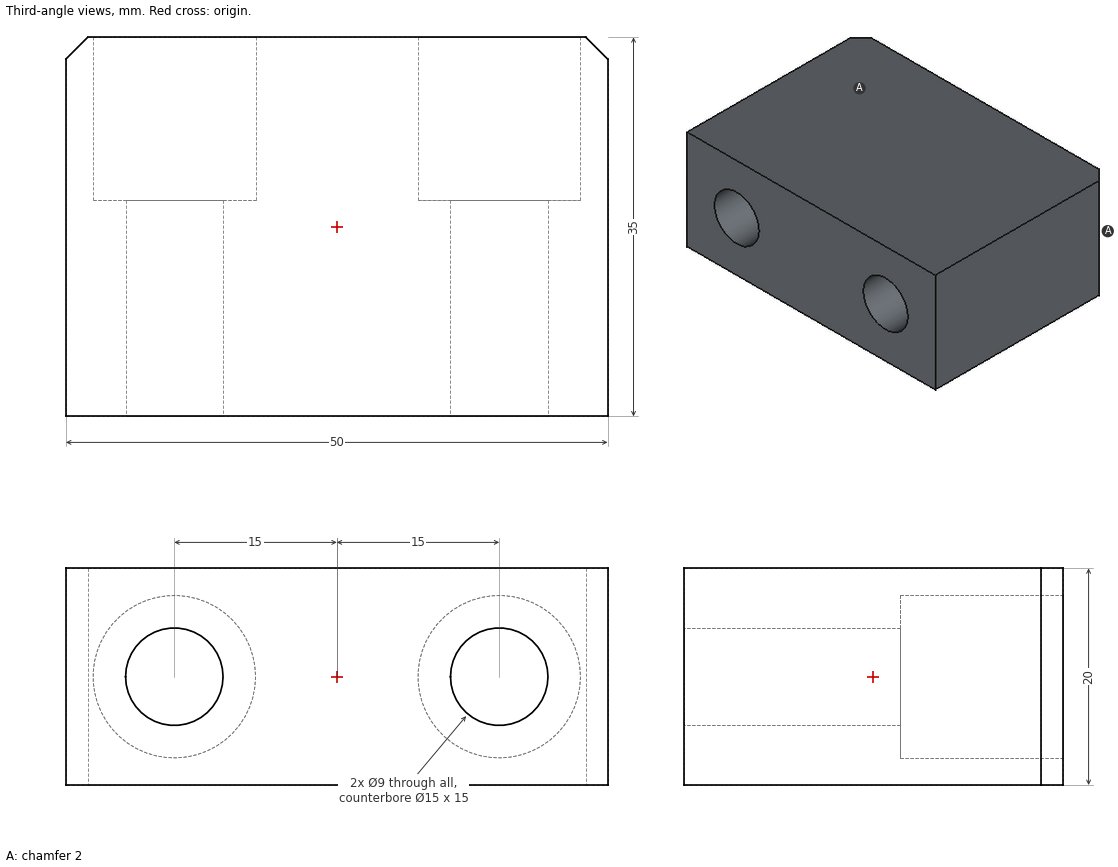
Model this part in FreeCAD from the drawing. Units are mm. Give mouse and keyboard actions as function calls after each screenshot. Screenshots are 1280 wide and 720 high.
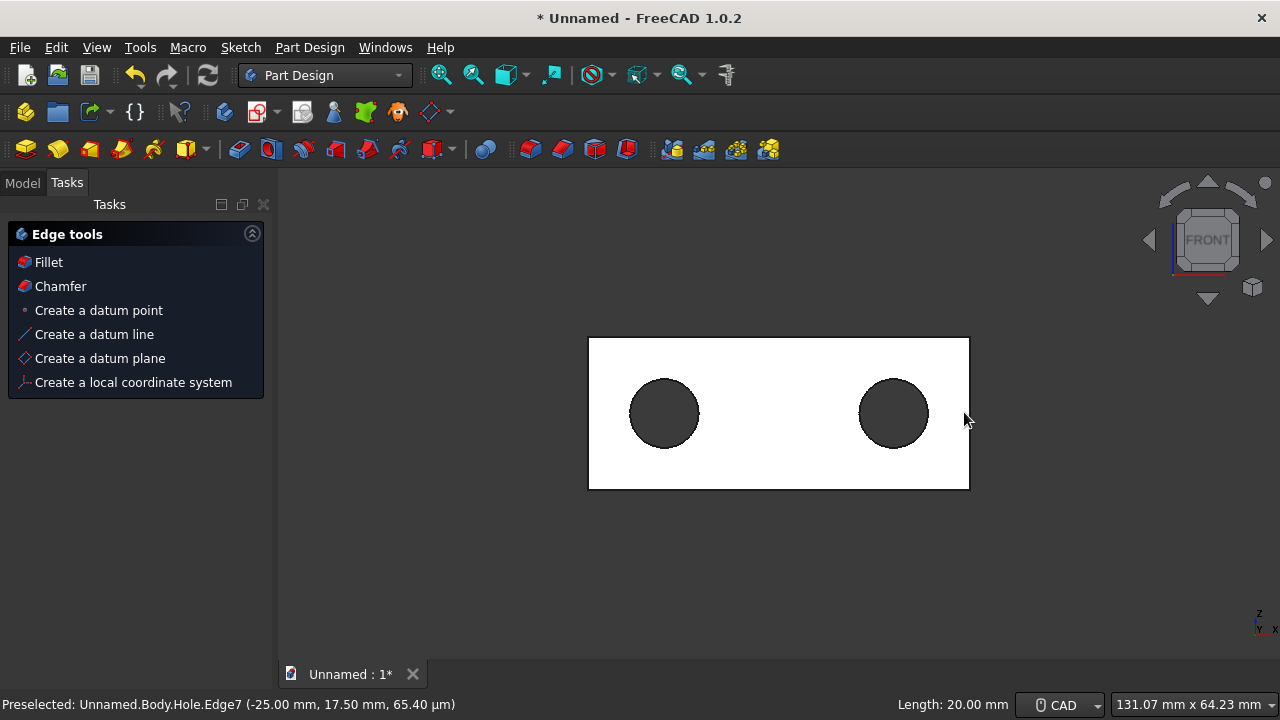
click(442, 76)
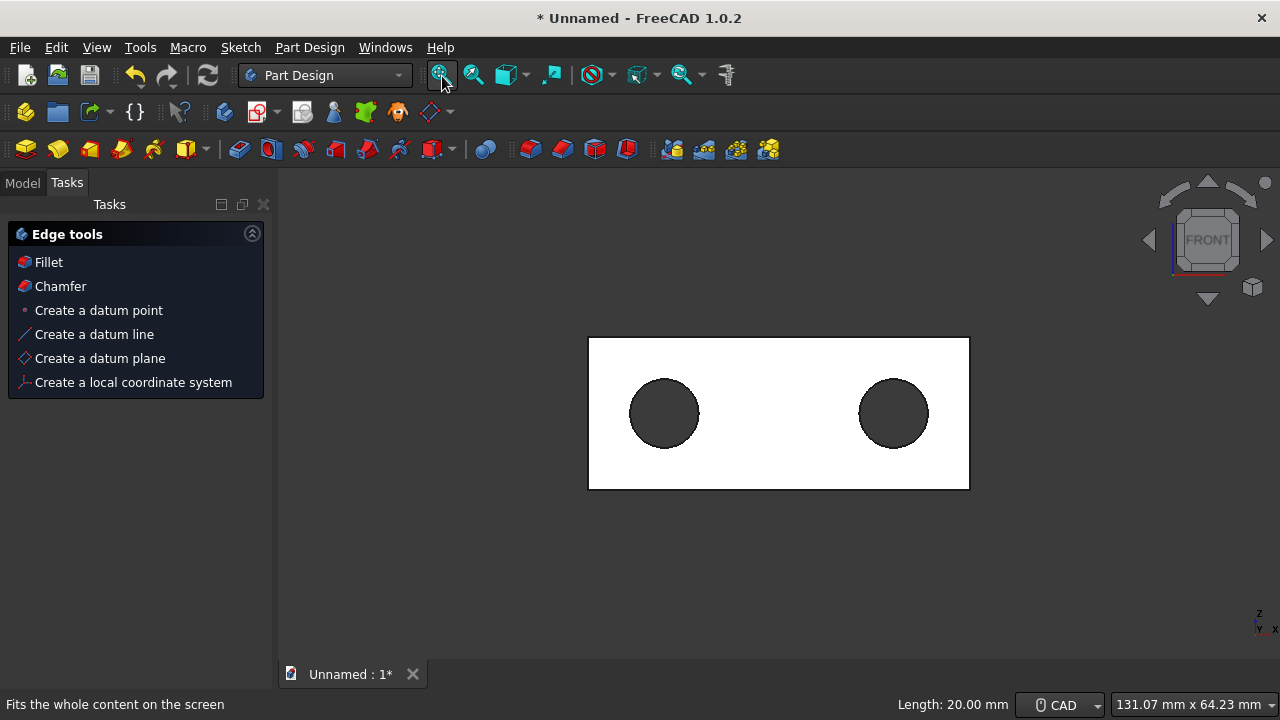
key(3)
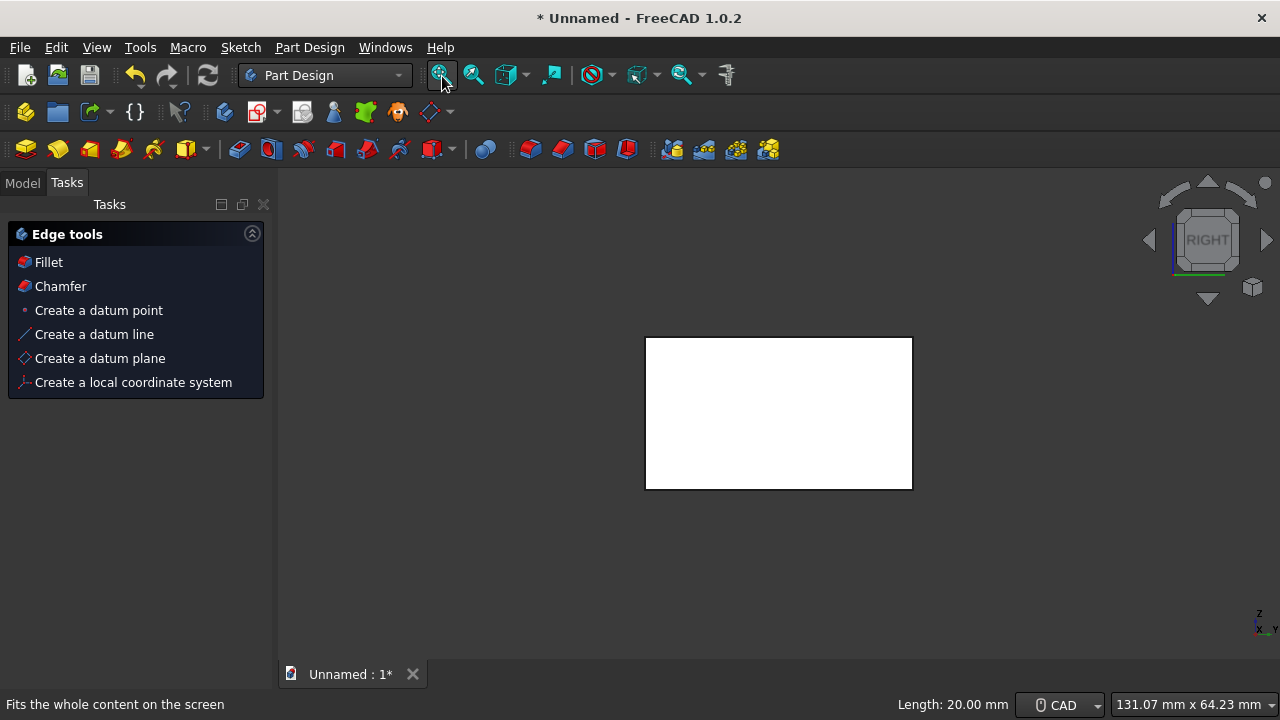
click(442, 76)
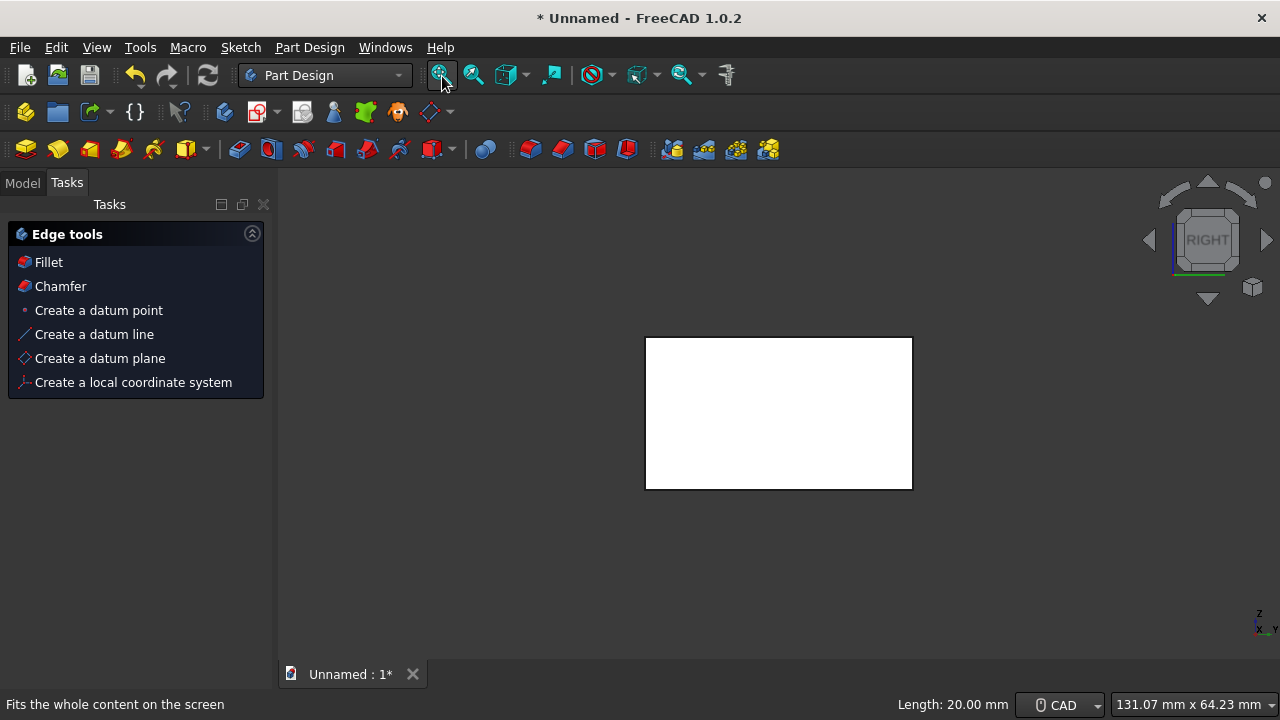
click(913, 412, ctrl)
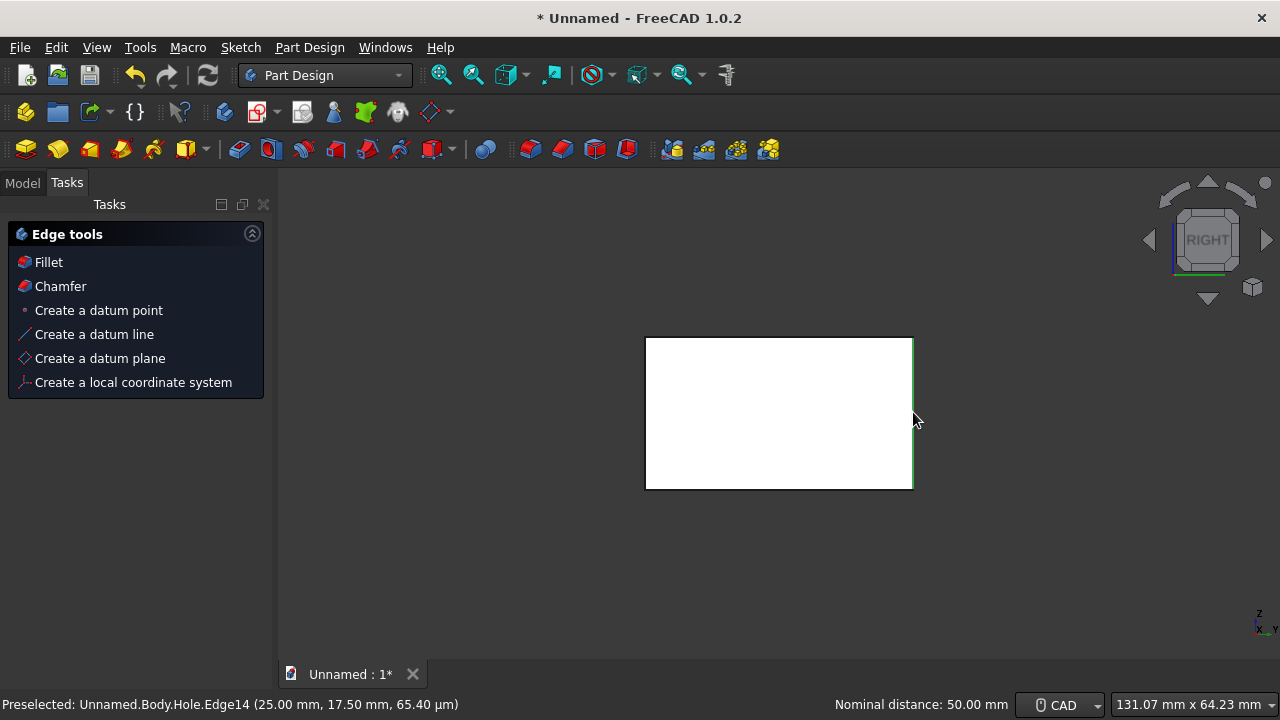
click(564, 150)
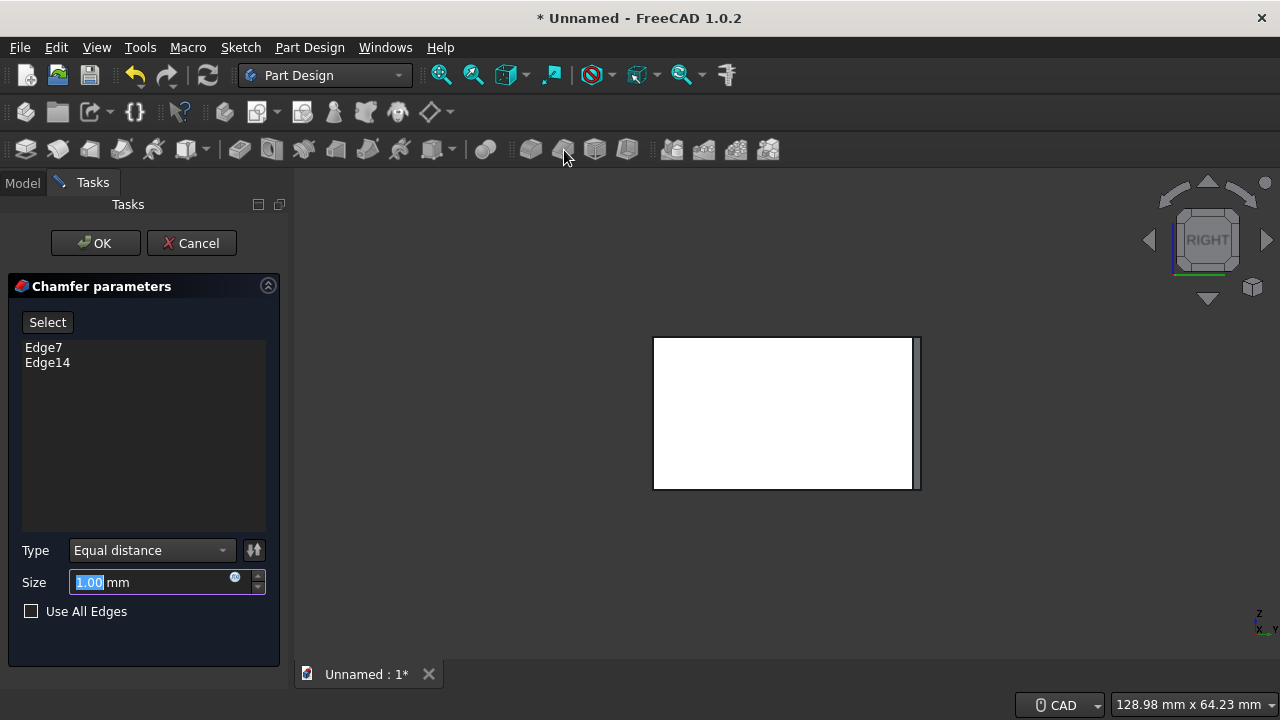
text(2)
key(Tab)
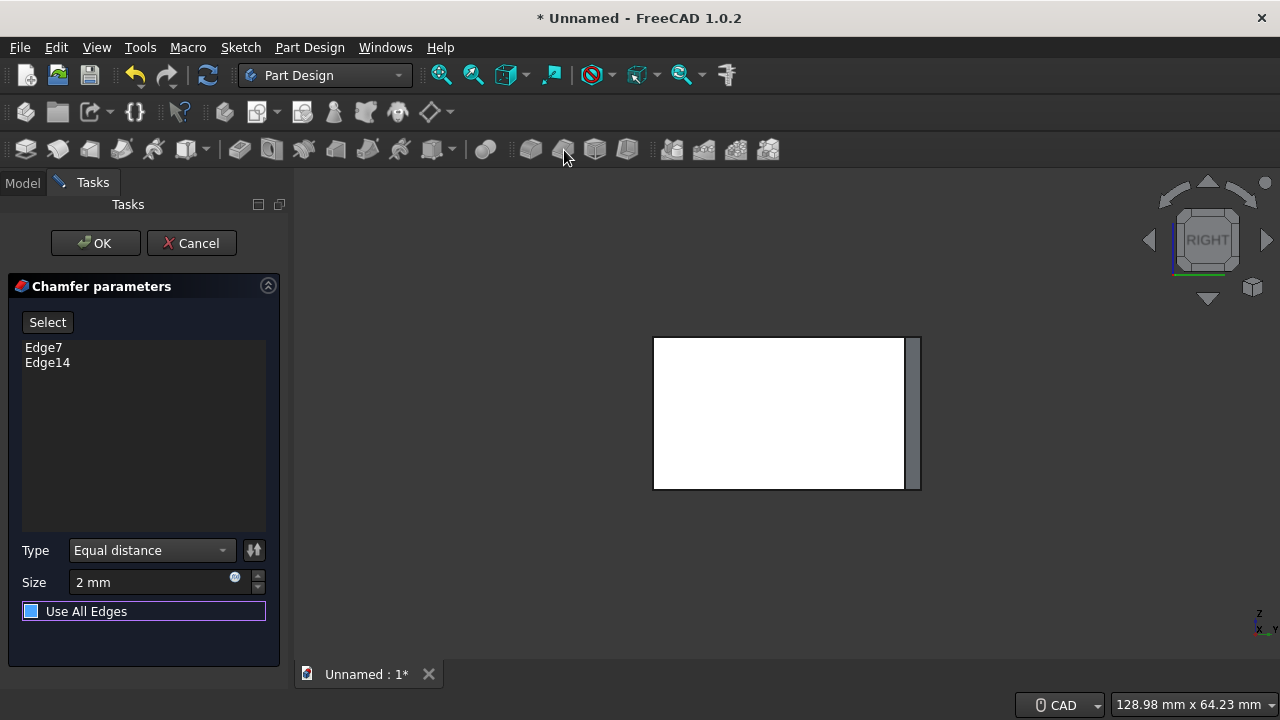
click(96, 243)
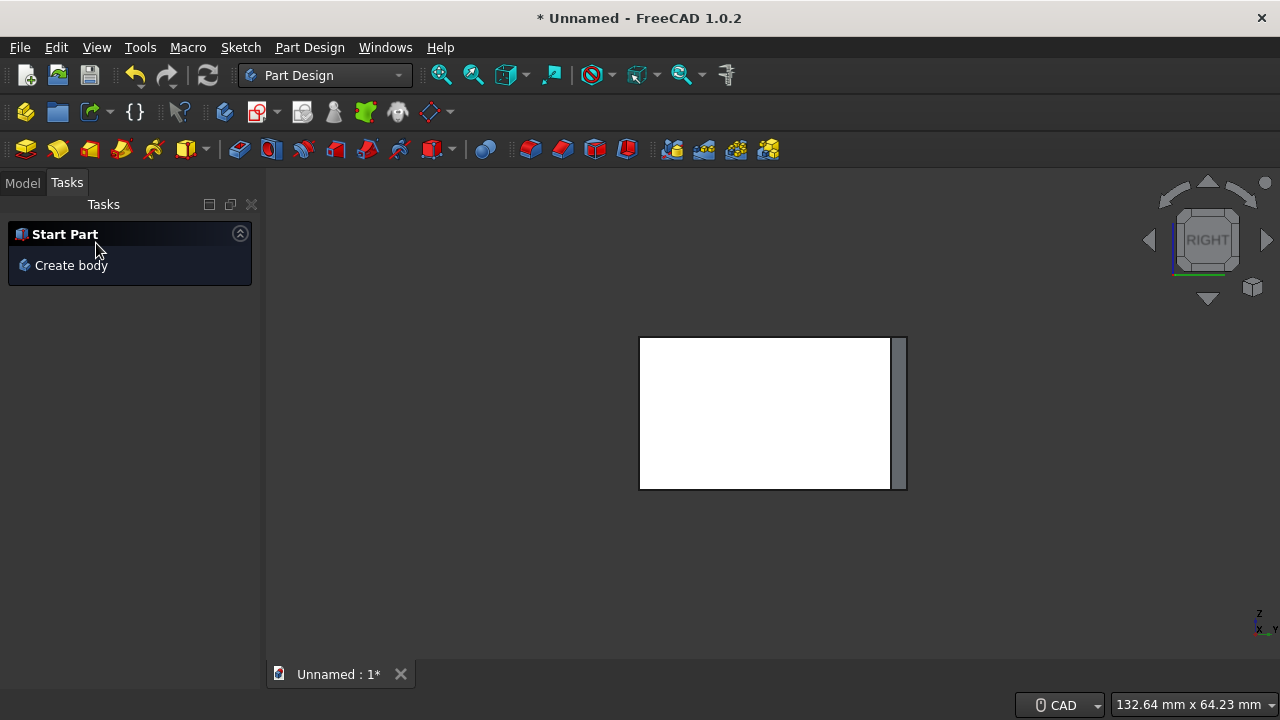
key(0)